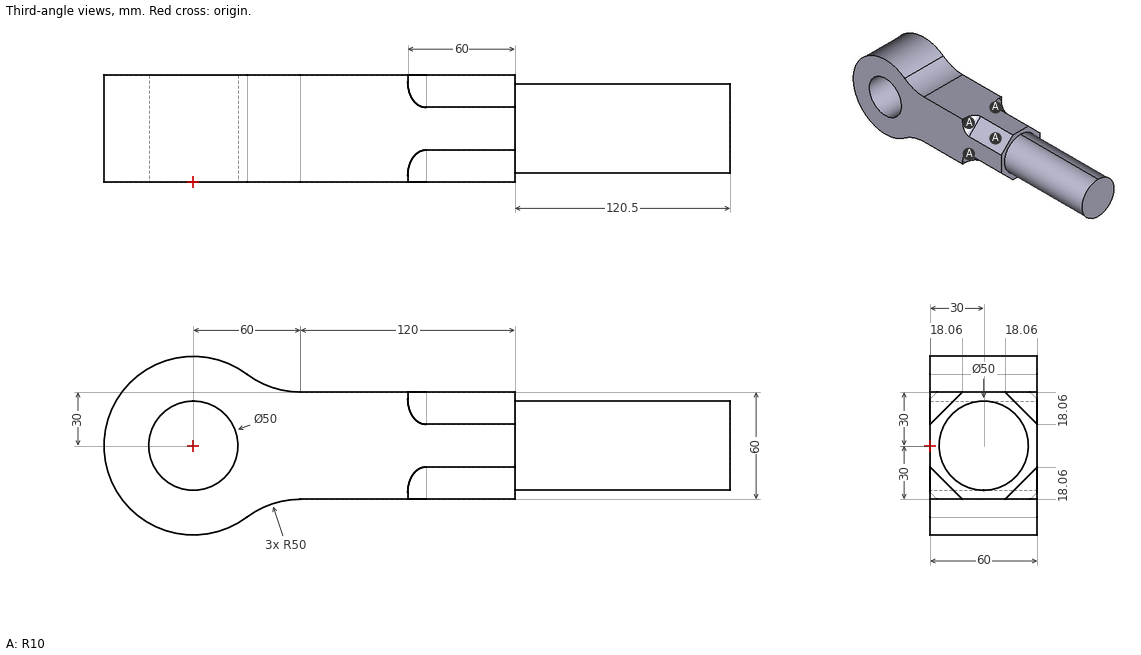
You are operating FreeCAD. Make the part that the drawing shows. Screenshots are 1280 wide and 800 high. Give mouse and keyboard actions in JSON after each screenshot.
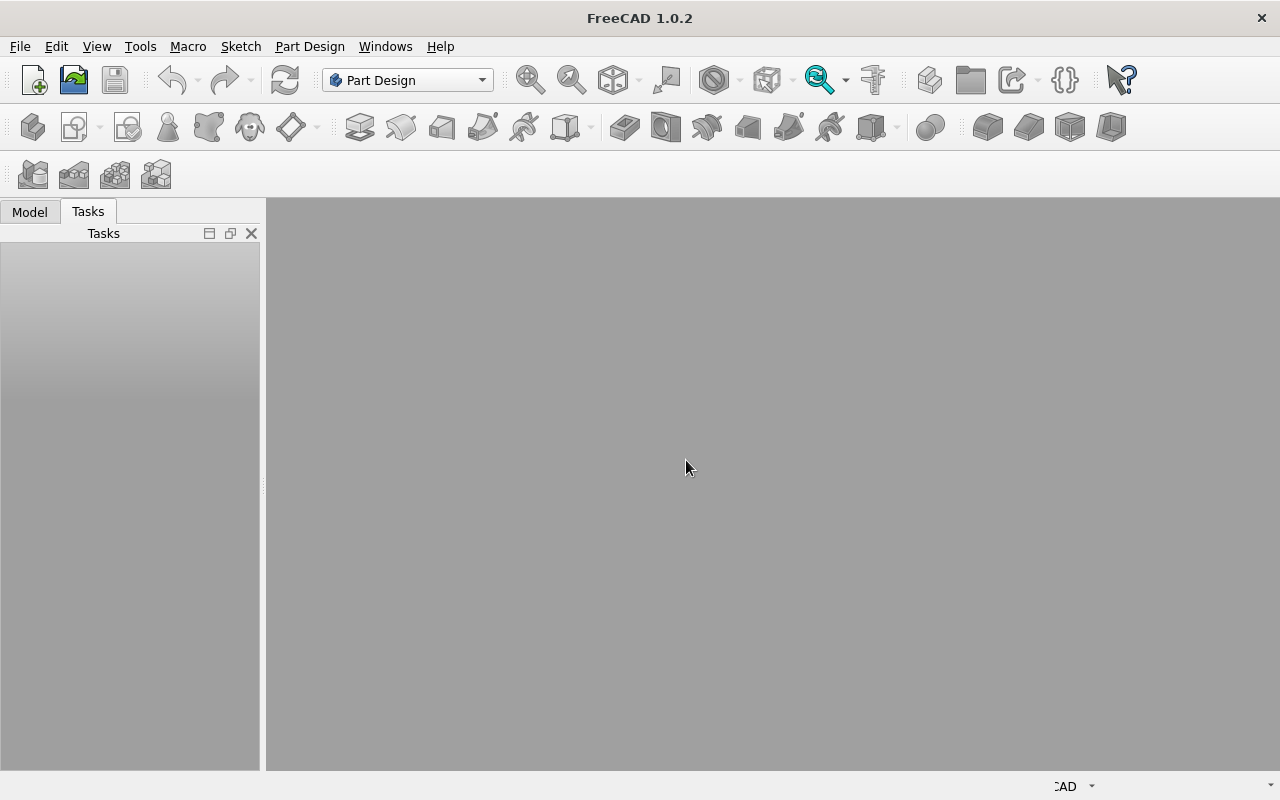
{"action": "key", "text": "ctrl+n"}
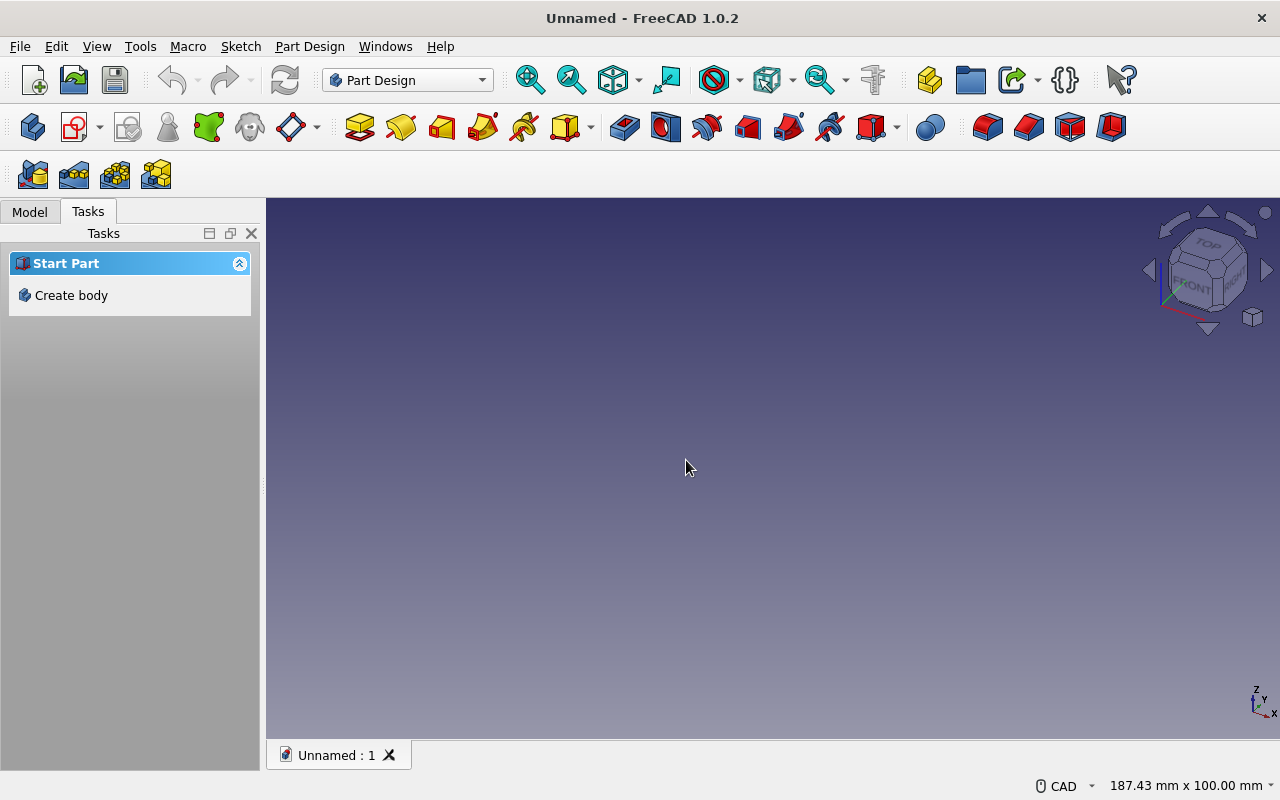
{"action": "left_click", "coordinate": [74, 128]}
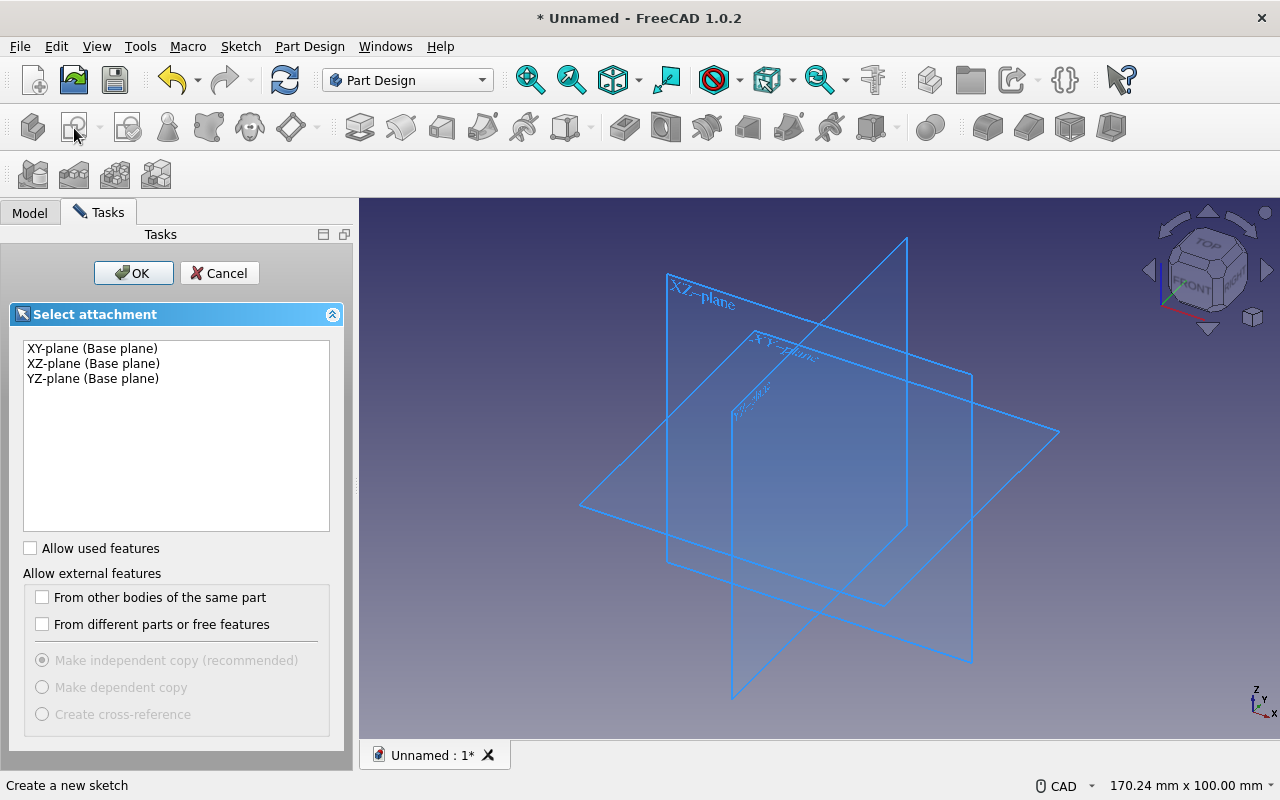
{"action": "left_click", "coordinate": [84, 364]}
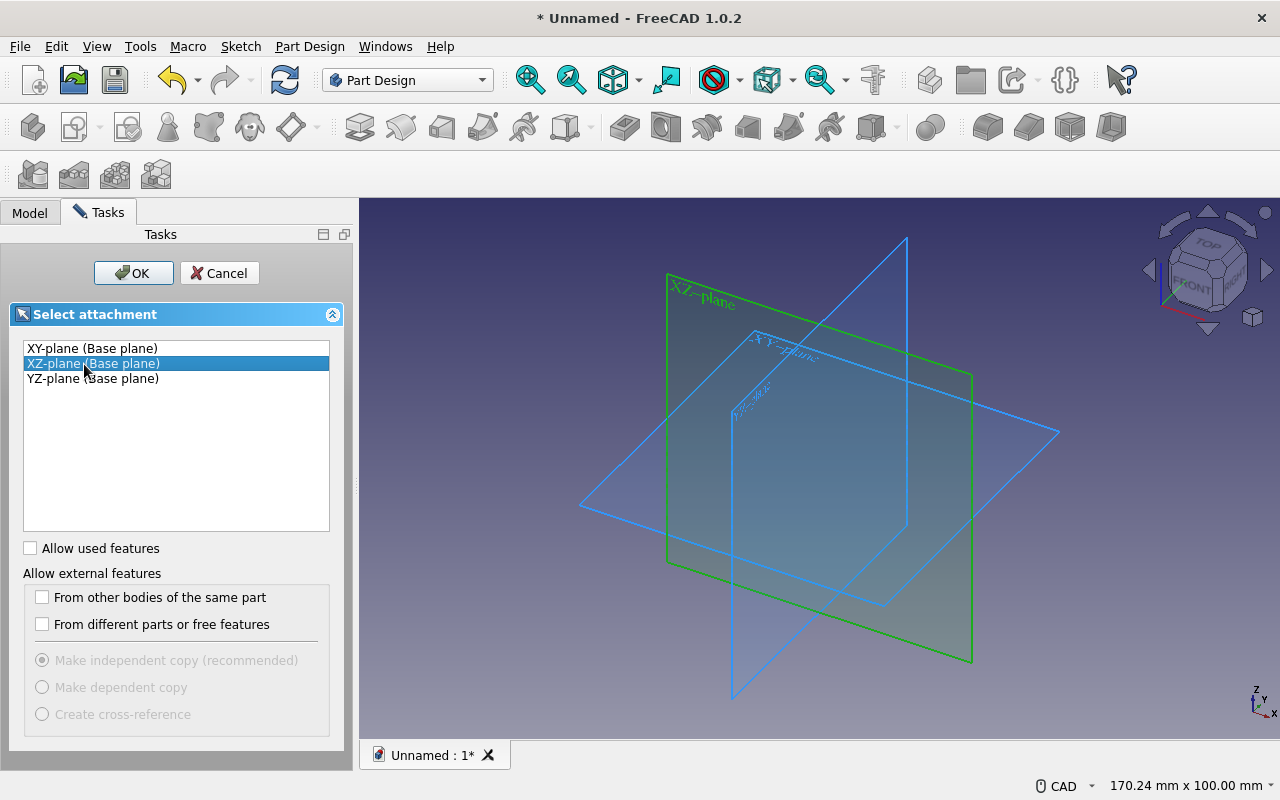
{"action": "left_click", "coordinate": [134, 273]}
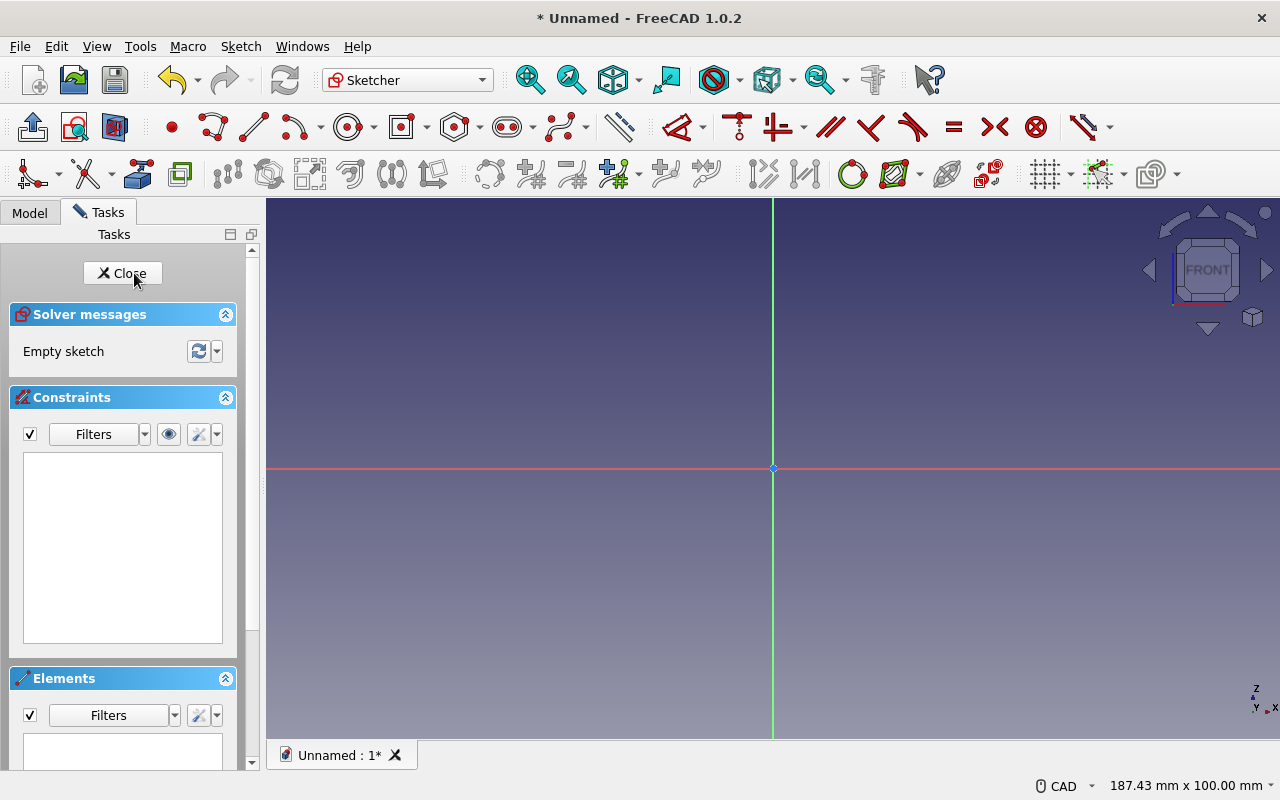
{"action": "scroll", "coordinate": [362, 469], "scroll_direction": "down", "scroll_amount": 4}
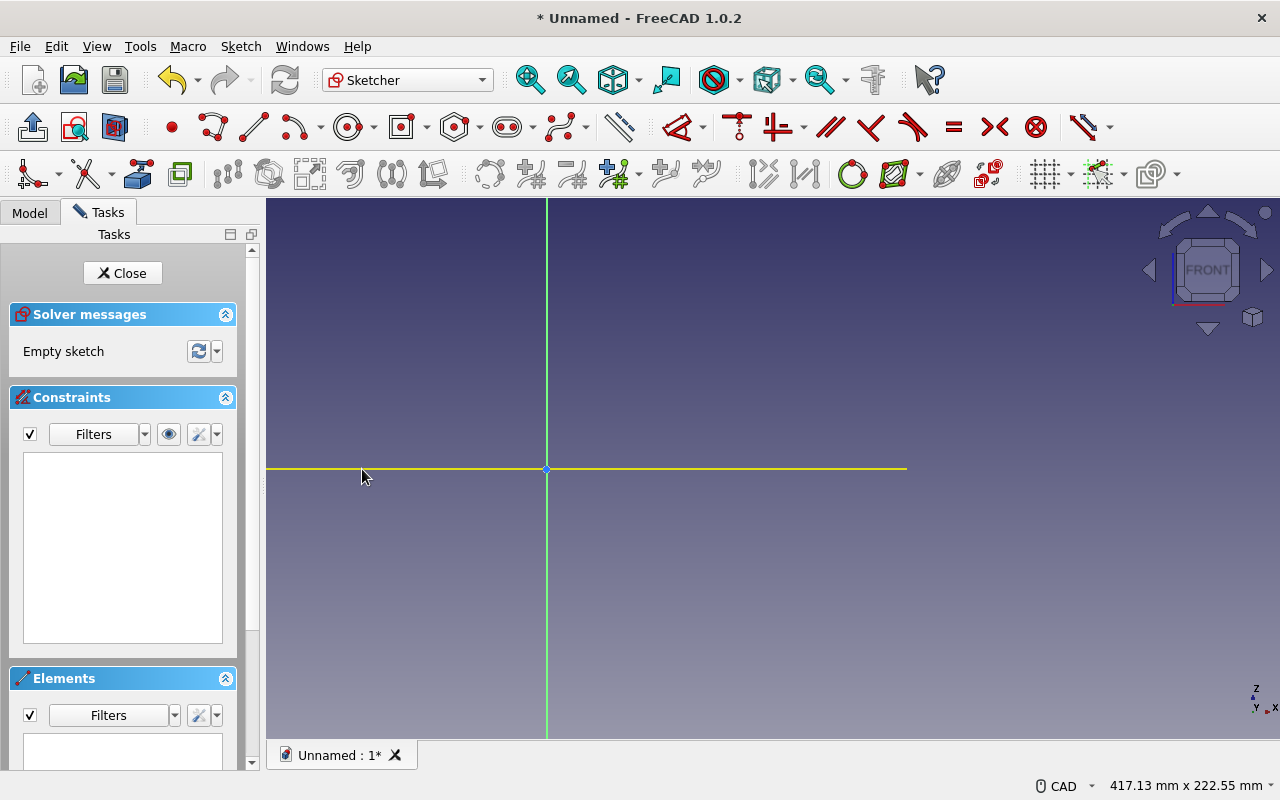
{"action": "key", "text": "g m"}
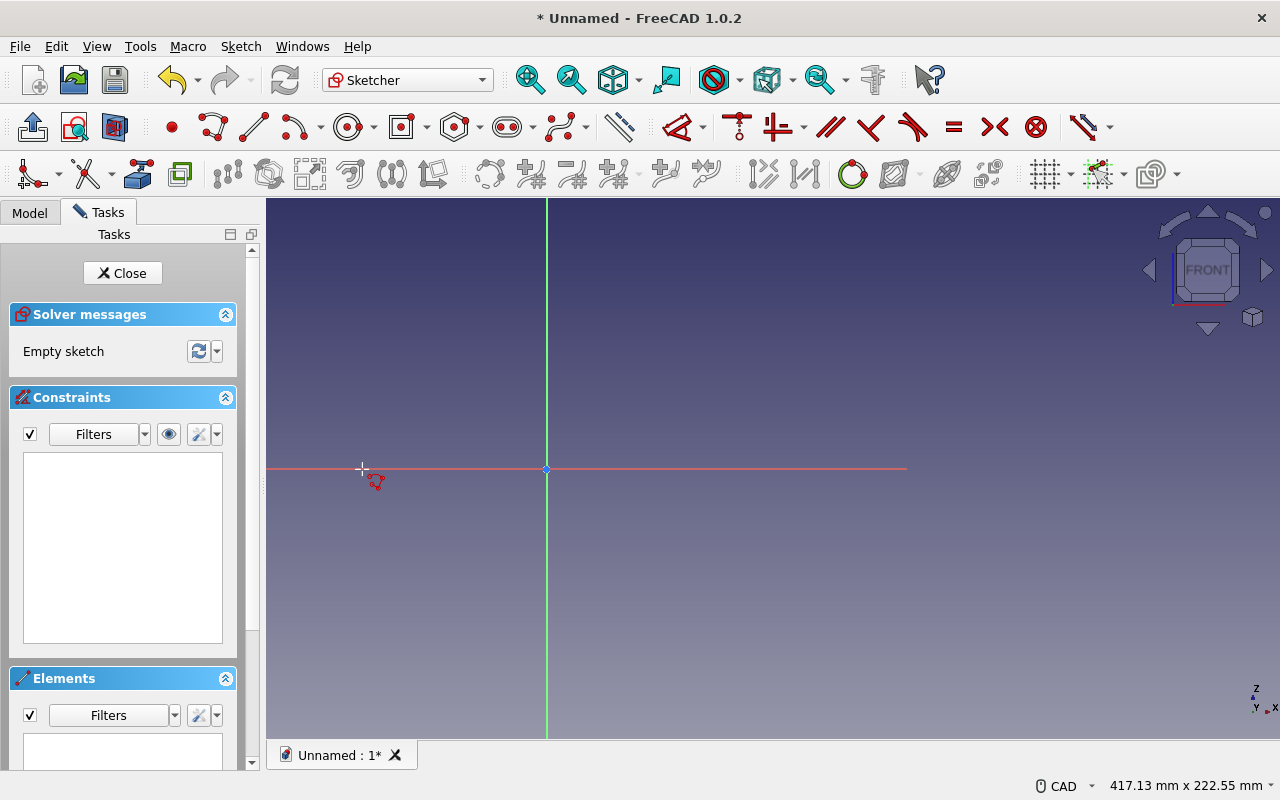
{"action": "left_click", "coordinate": [693, 396]}
{"action": "left_click", "coordinate": [984, 396]}
{"action": "left_click", "coordinate": [984, 542]}
{"action": "left_click", "coordinate": [693, 542]}
{"action": "right_click", "coordinate": [693, 542]}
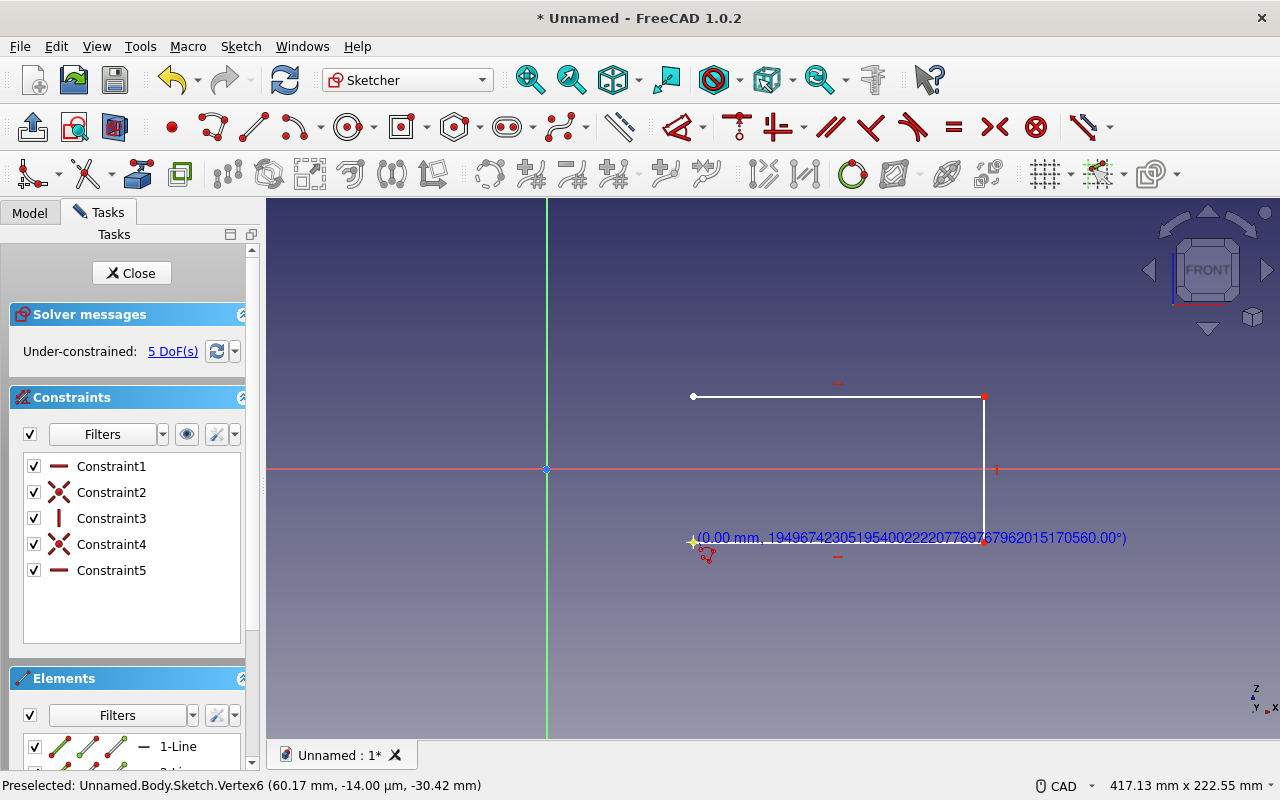
{"action": "key", "text": "g 3 a"}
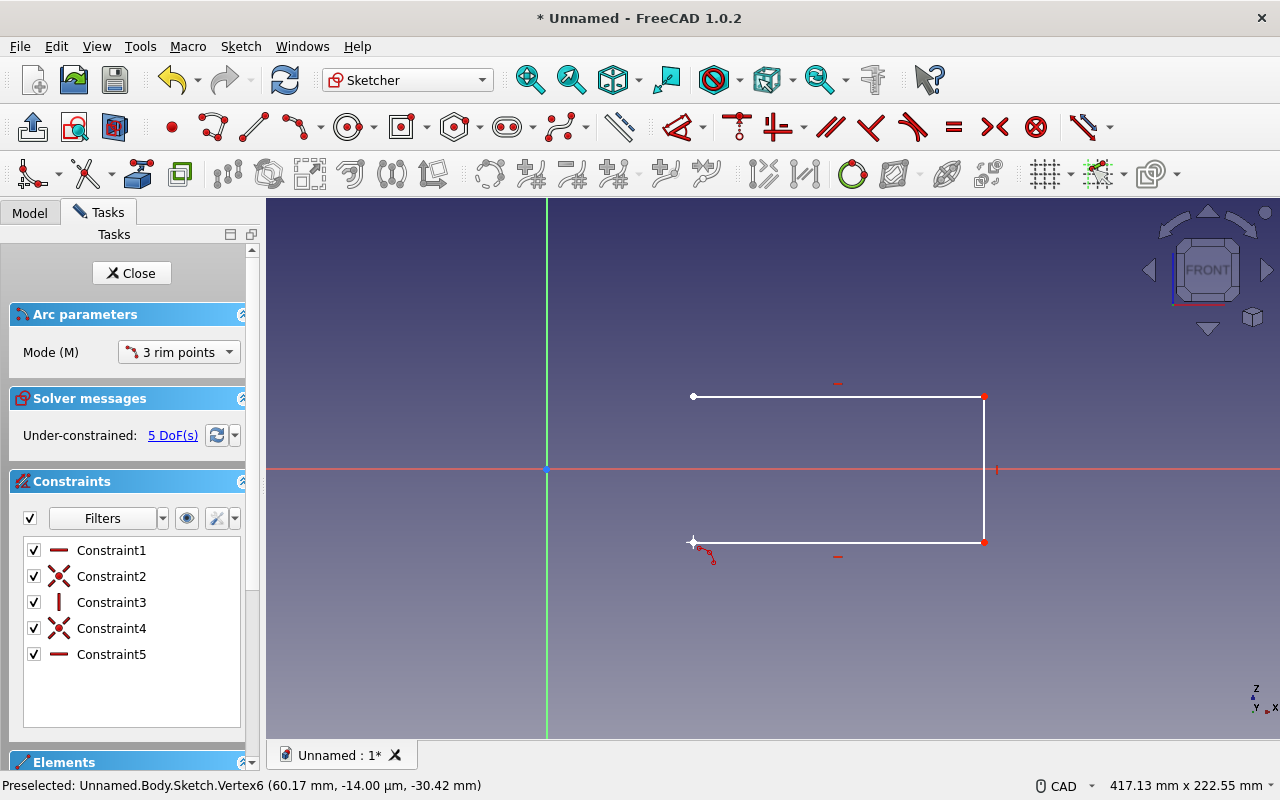
{"action": "left_click", "coordinate": [693, 543]}
{"action": "left_click", "coordinate": [620, 566]}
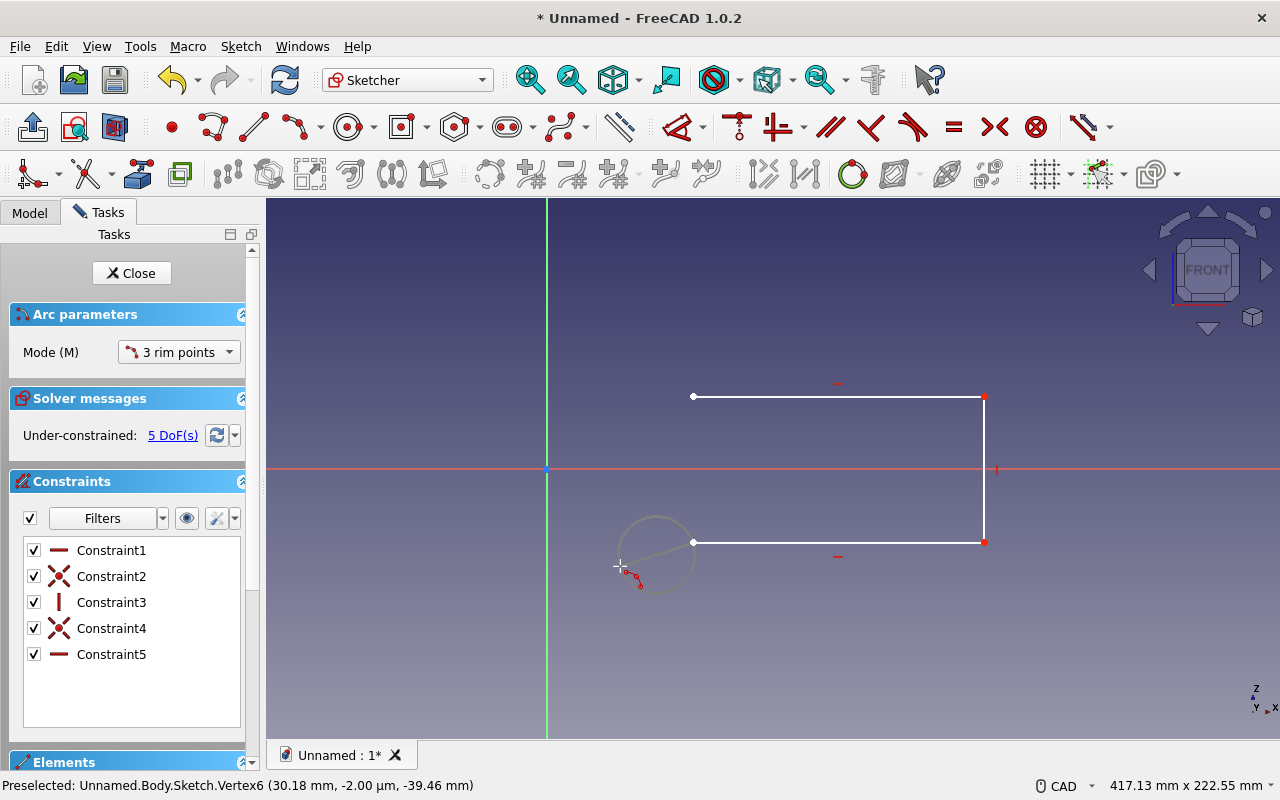
{"action": "scroll", "coordinate": [654, 548], "scroll_direction": "up", "scroll_amount": 5}